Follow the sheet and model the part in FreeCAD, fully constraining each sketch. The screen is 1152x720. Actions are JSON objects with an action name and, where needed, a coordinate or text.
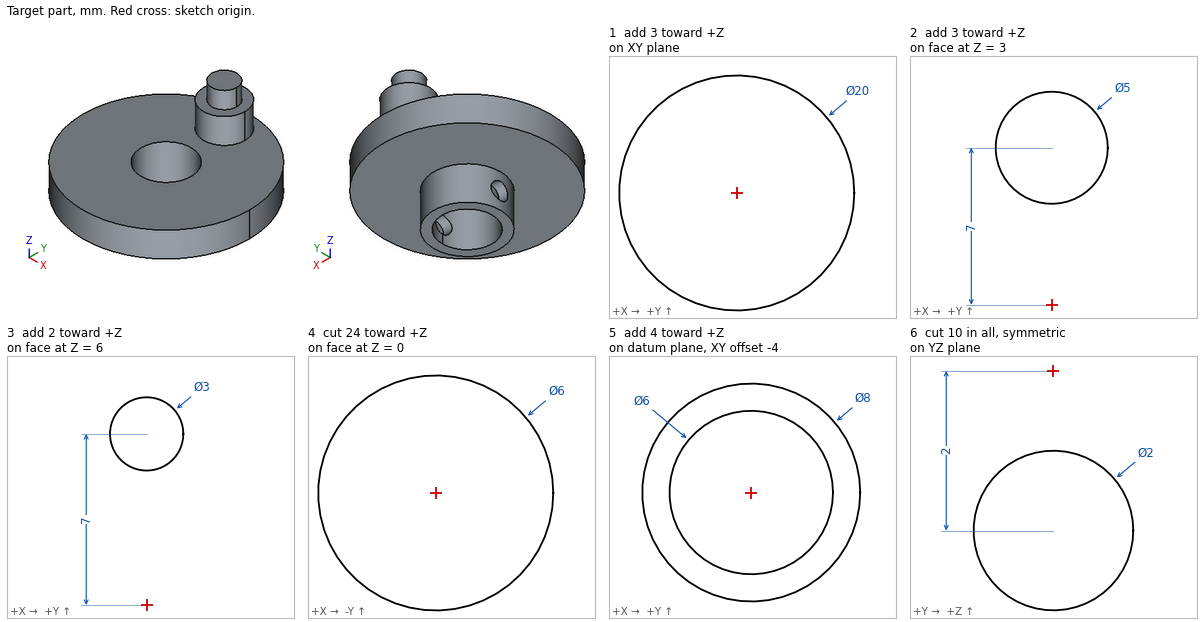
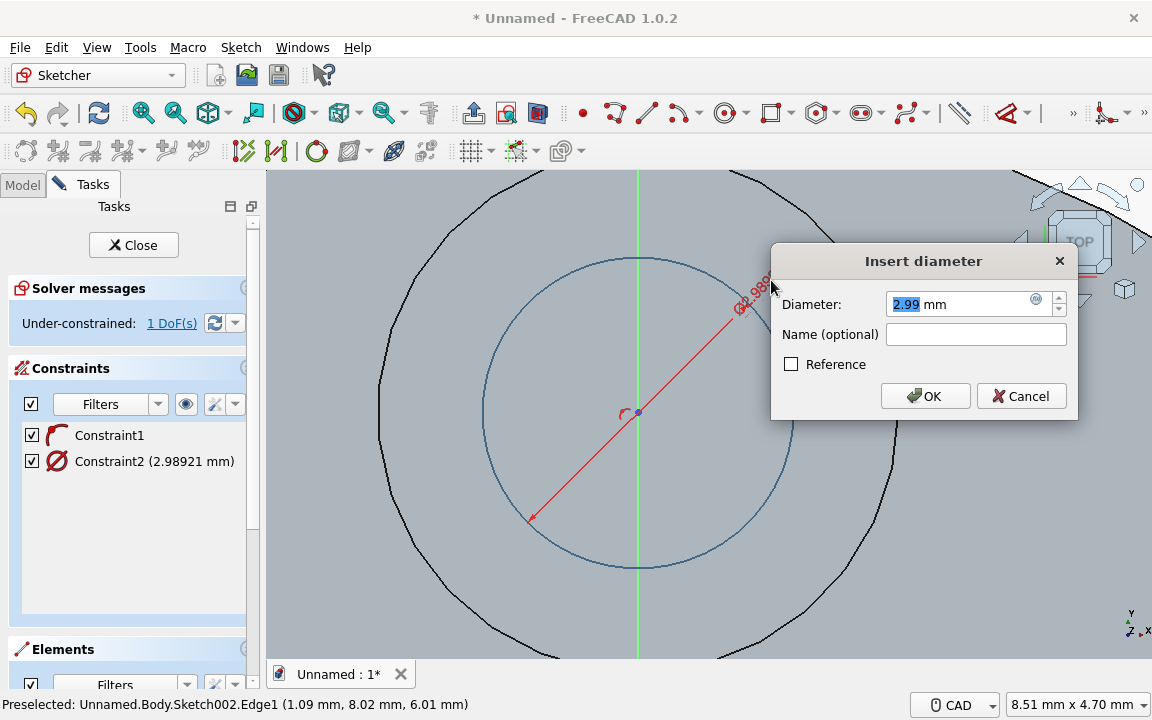
{"action": "type", "text": "3"}
{"action": "key", "text": "Return"}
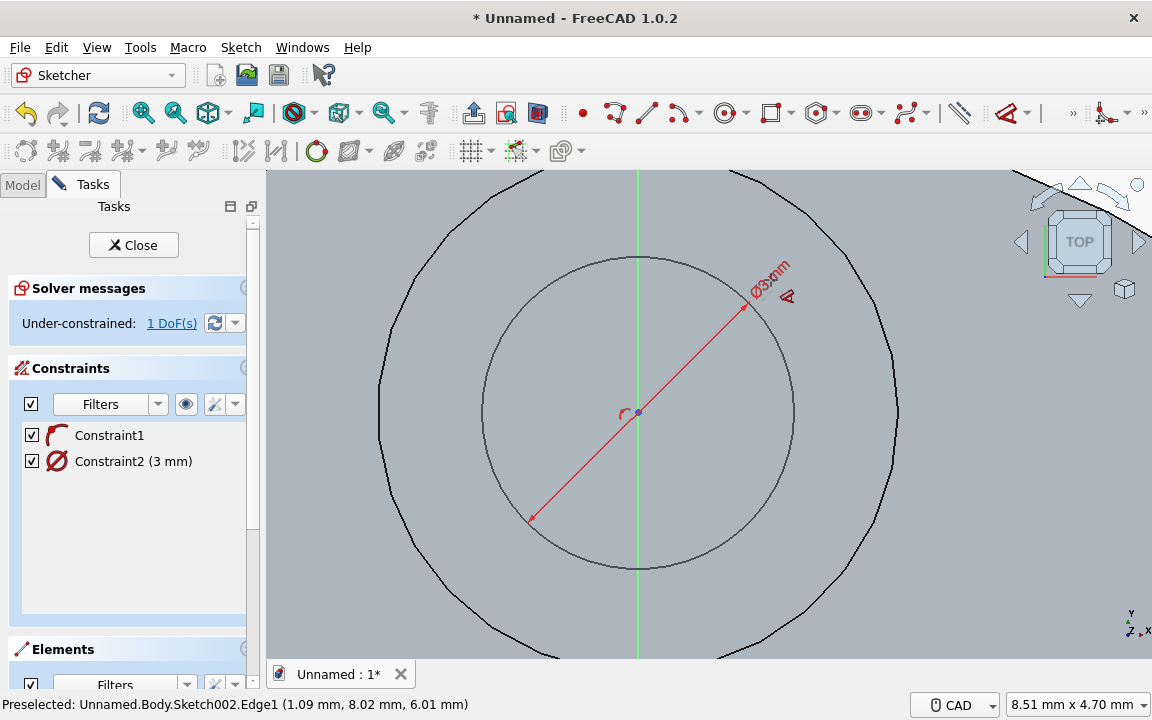
{"action": "left_click", "coordinate": [638, 413]}
{"action": "left_click", "coordinate": [672, 522]}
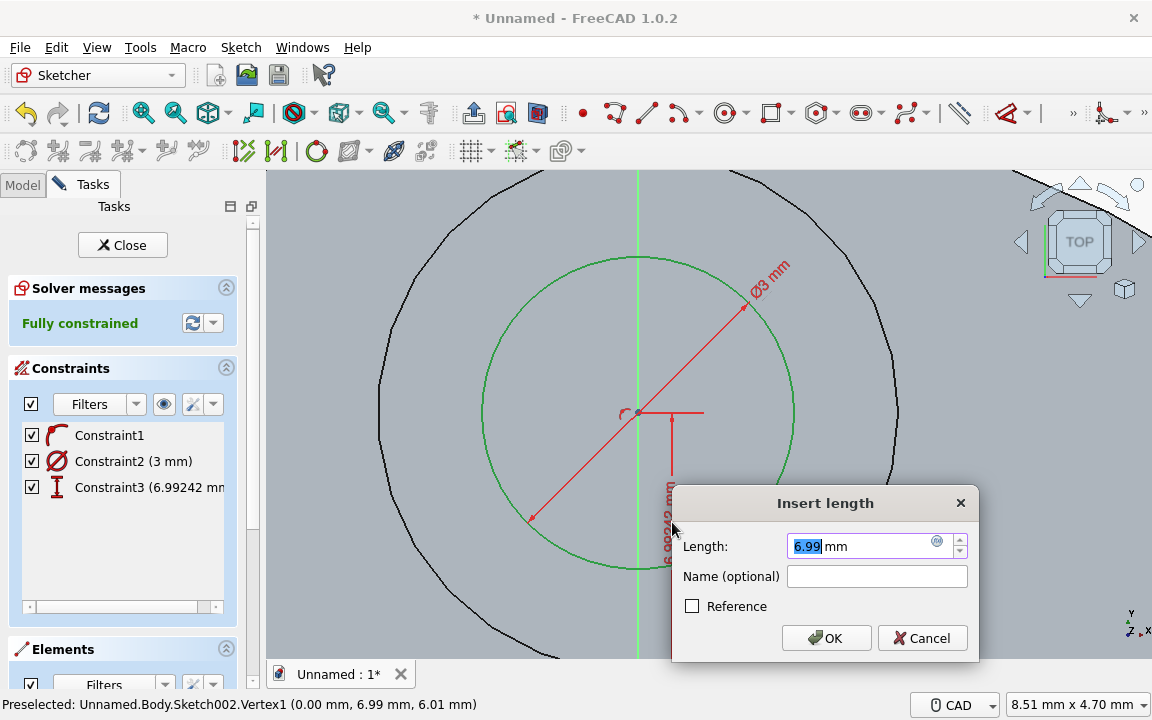
{"action": "type", "text": "7"}
{"action": "key", "text": "Return"}
{"action": "key", "text": "Escape"}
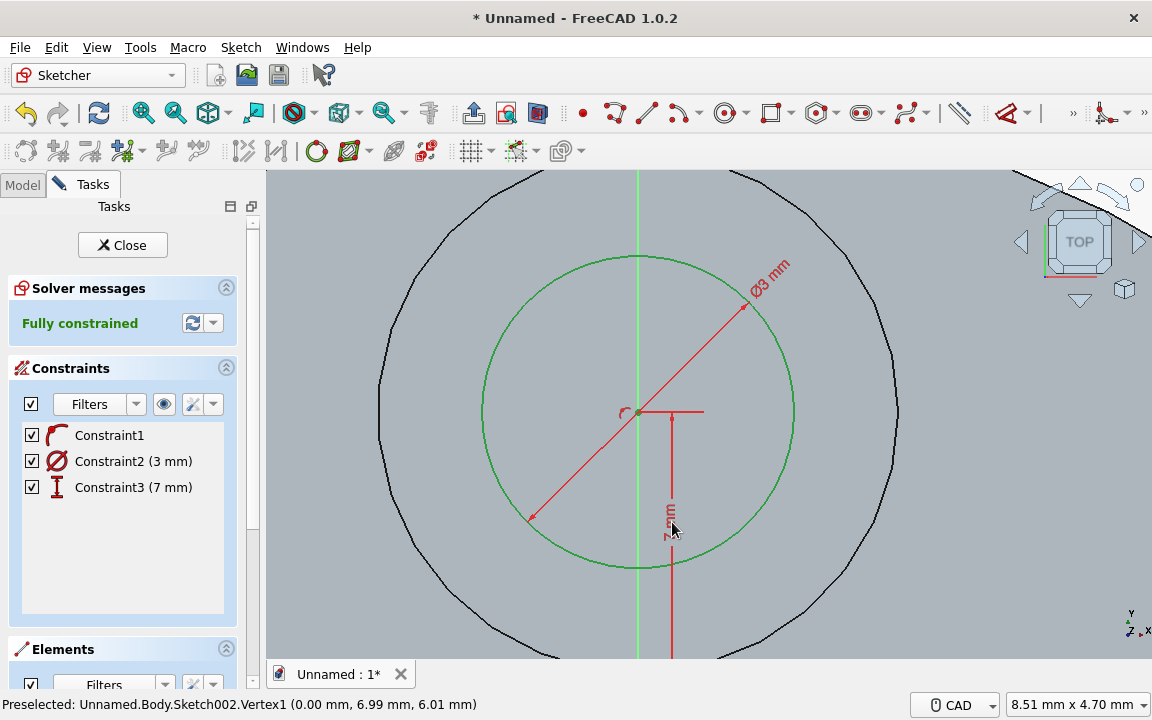
{"action": "left_click", "coordinate": [123, 245]}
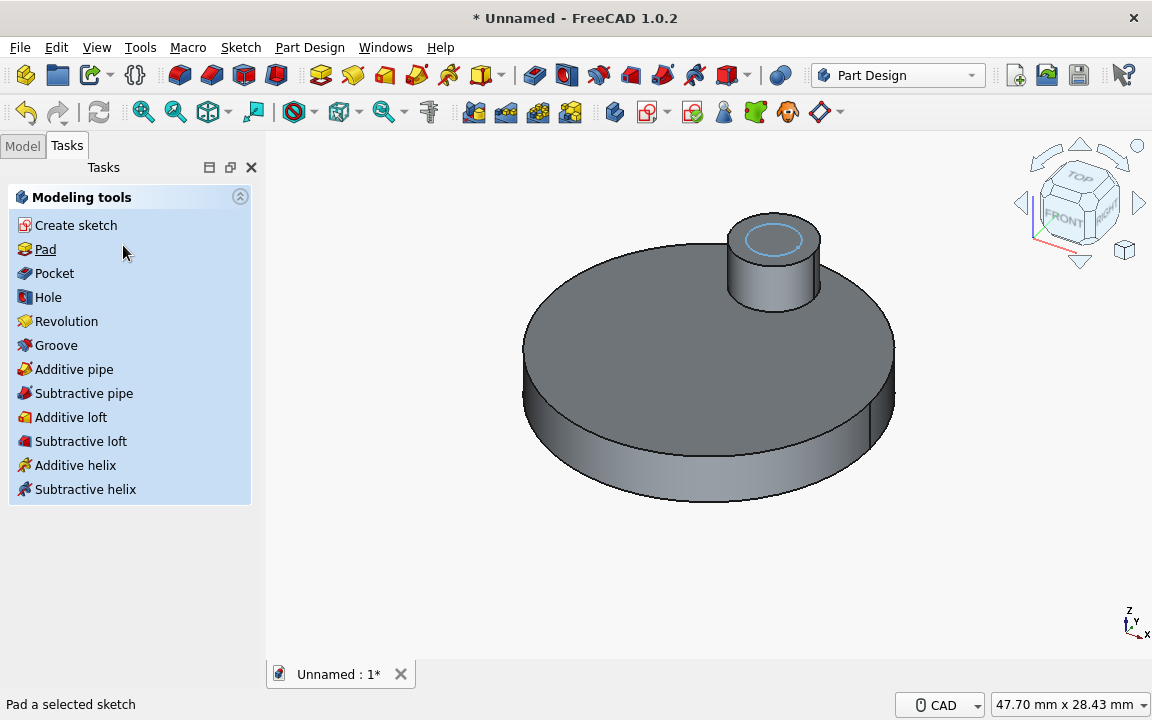
{"action": "left_click", "coordinate": [322, 76]}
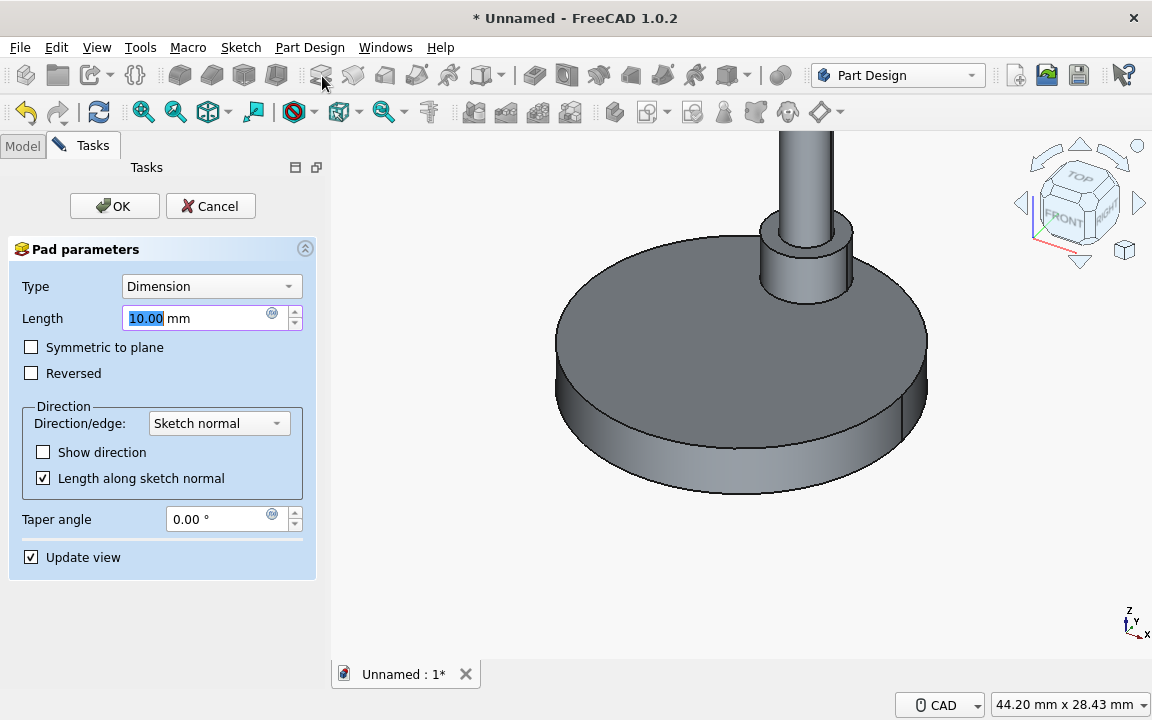
{"action": "type", "text": "2"}
{"action": "key", "text": "Tab"}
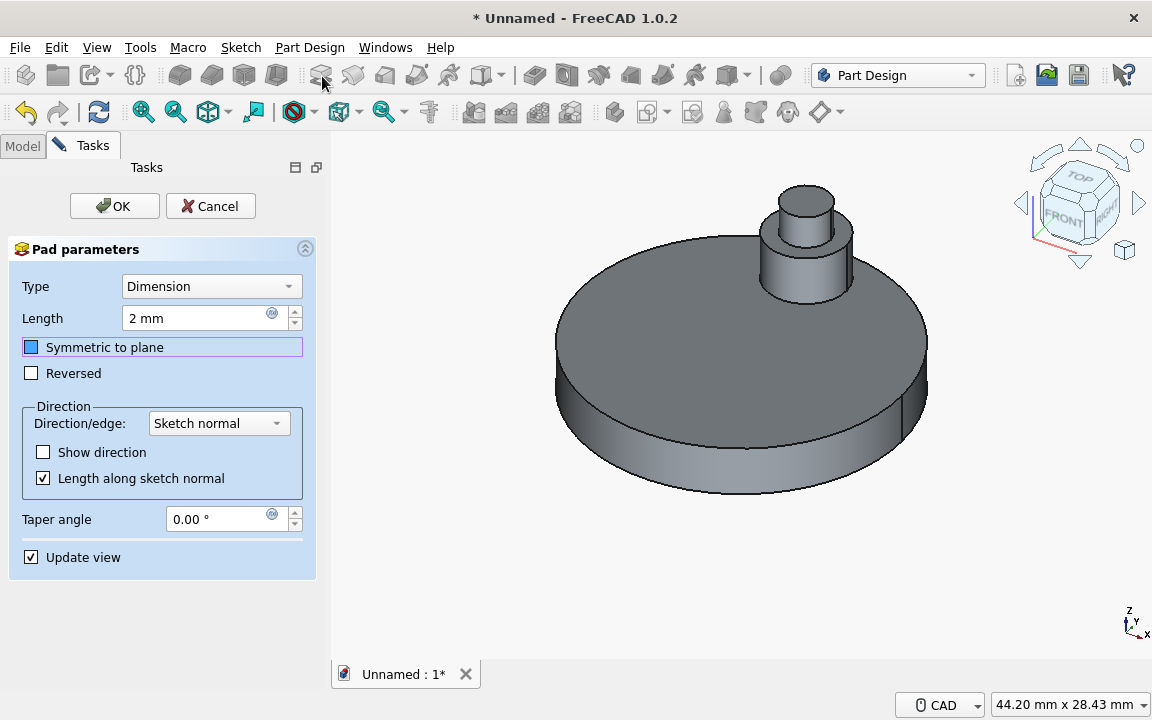
{"action": "left_click", "coordinate": [115, 206]}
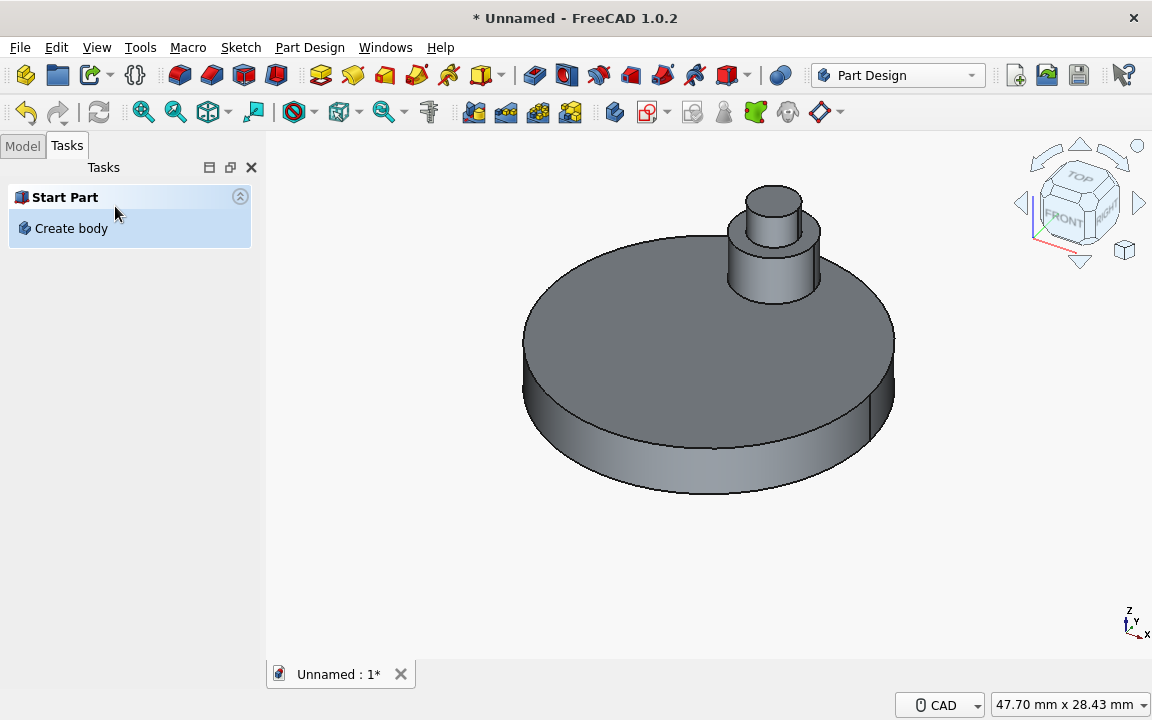
{"action": "left_click", "coordinate": [144, 112]}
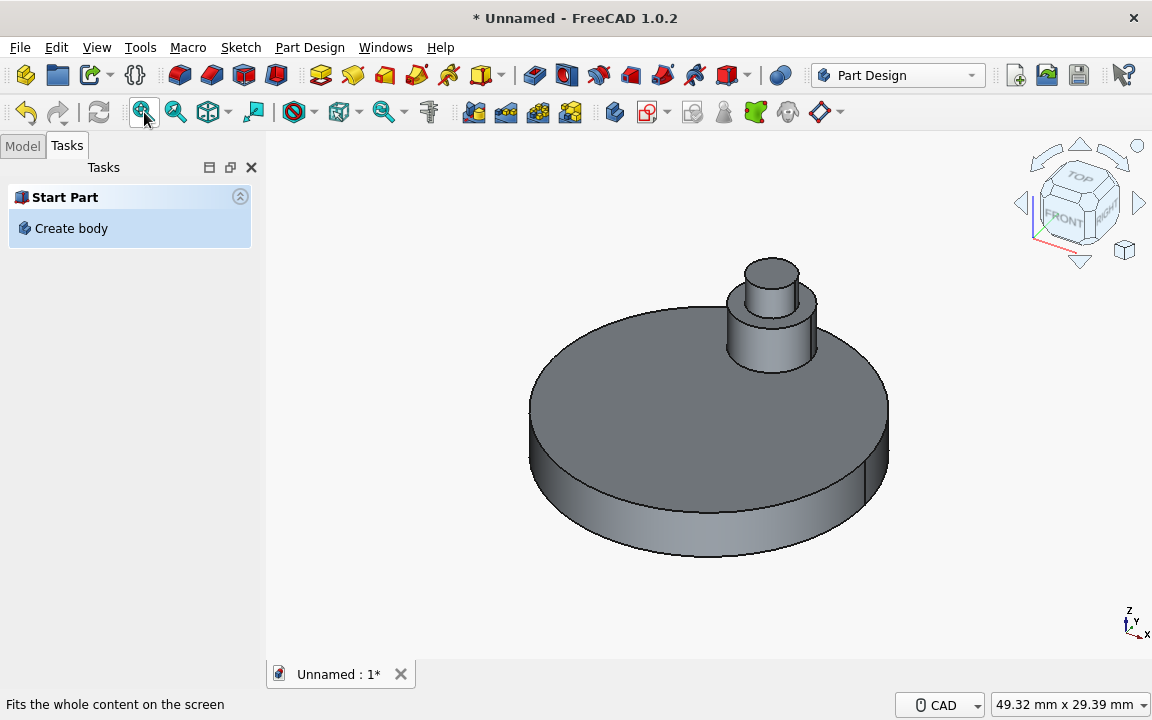
{"action": "key", "text": "5"}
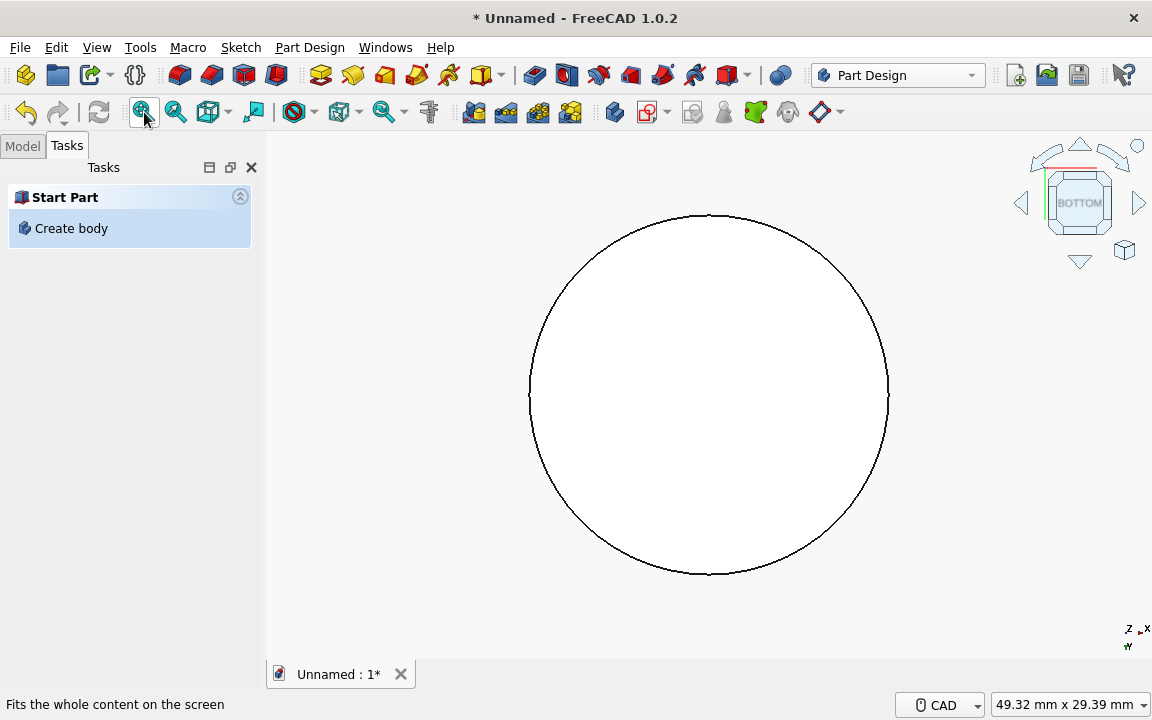
{"action": "left_click", "coordinate": [709, 394]}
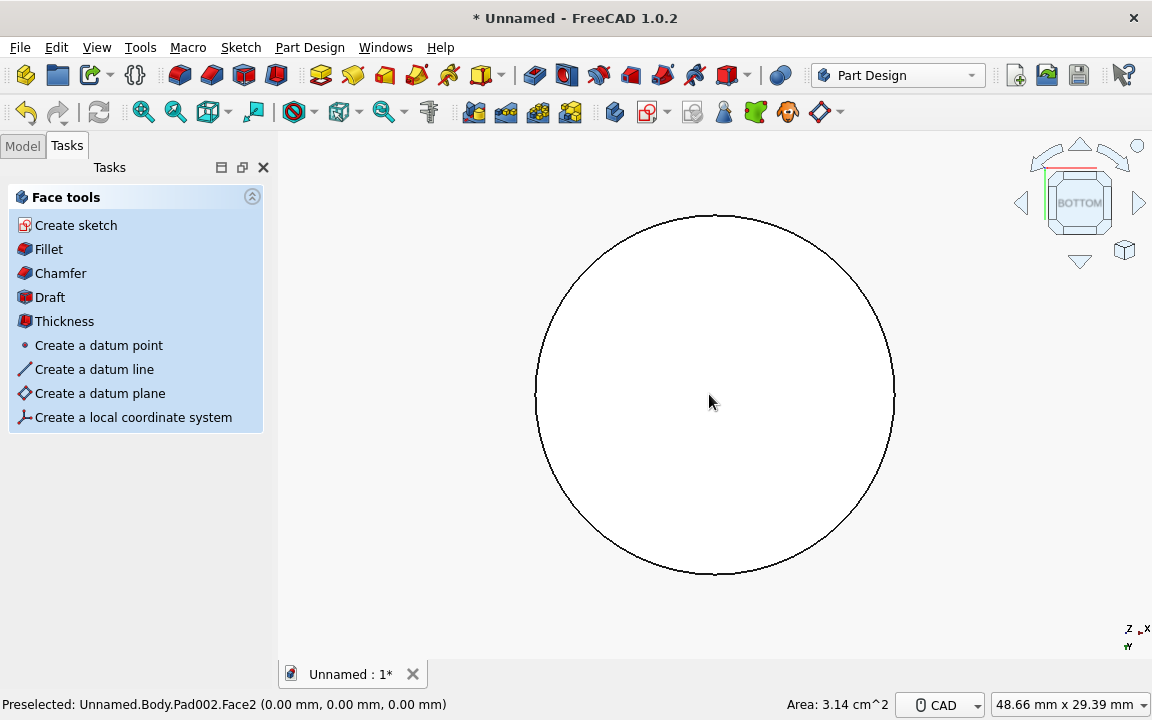
{"action": "left_click", "coordinate": [648, 112]}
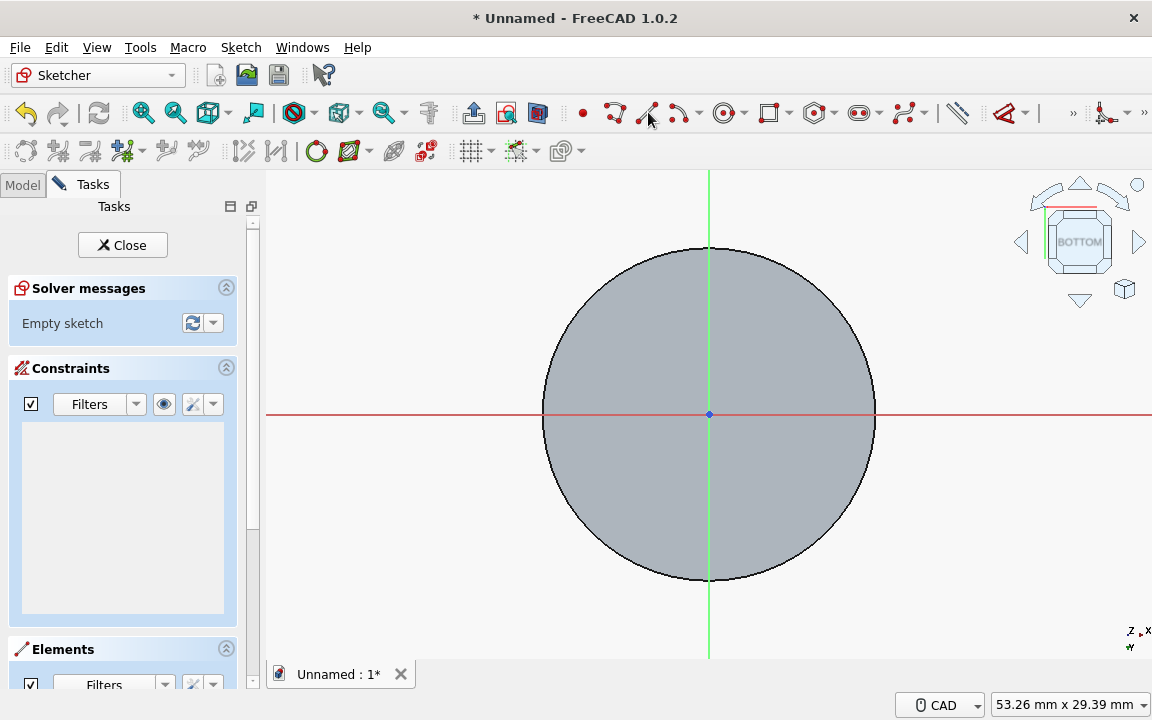
{"action": "scroll", "coordinate": [739, 415], "scroll_direction": "up", "scroll_amount": 6}